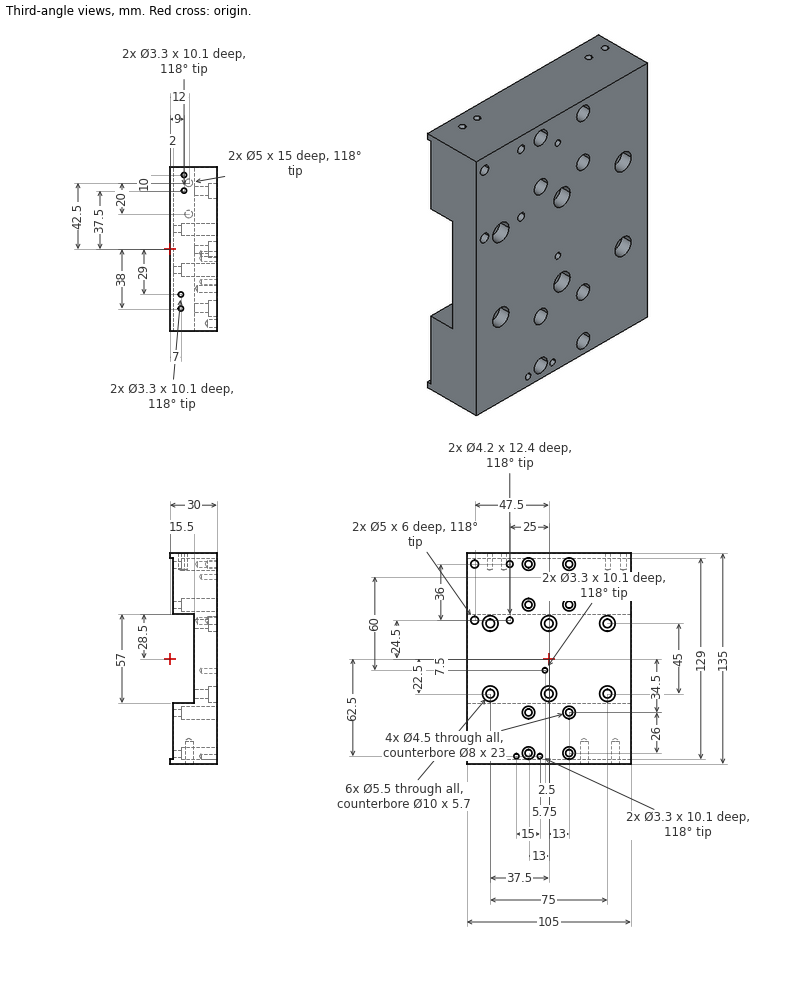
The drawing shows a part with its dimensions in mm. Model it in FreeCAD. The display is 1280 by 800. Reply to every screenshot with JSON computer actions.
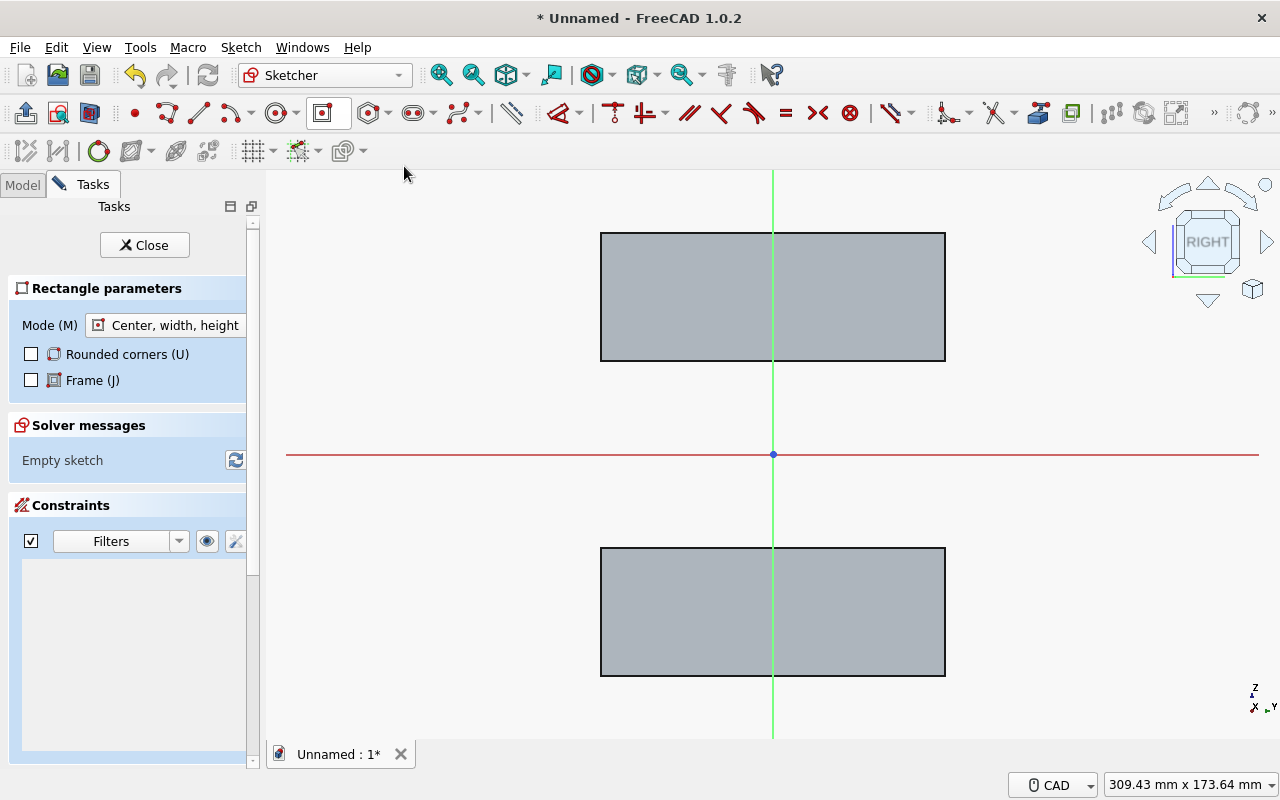
{"action": "left_click", "coordinate": [773, 454]}
{"action": "left_click", "coordinate": [945, 243]}
{"action": "key", "text": "Escape"}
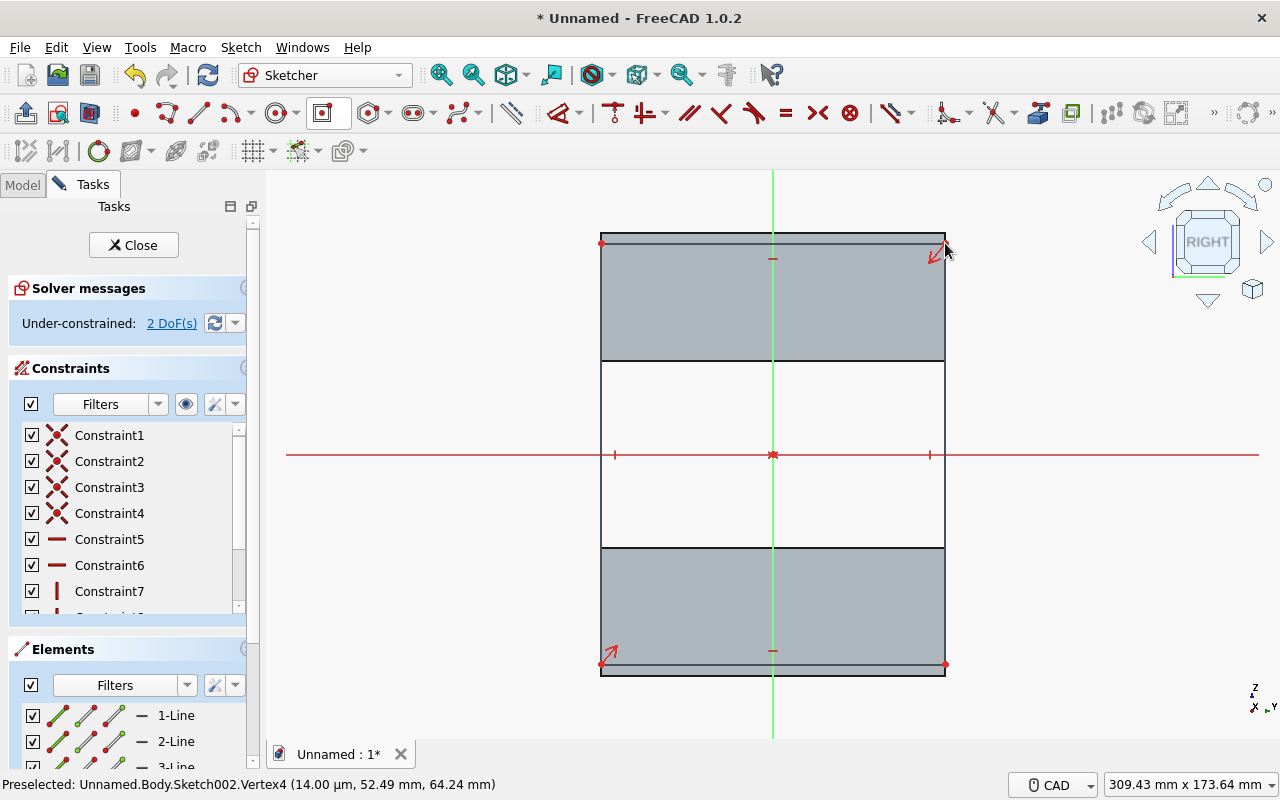
{"action": "left_click", "coordinate": [558, 114]}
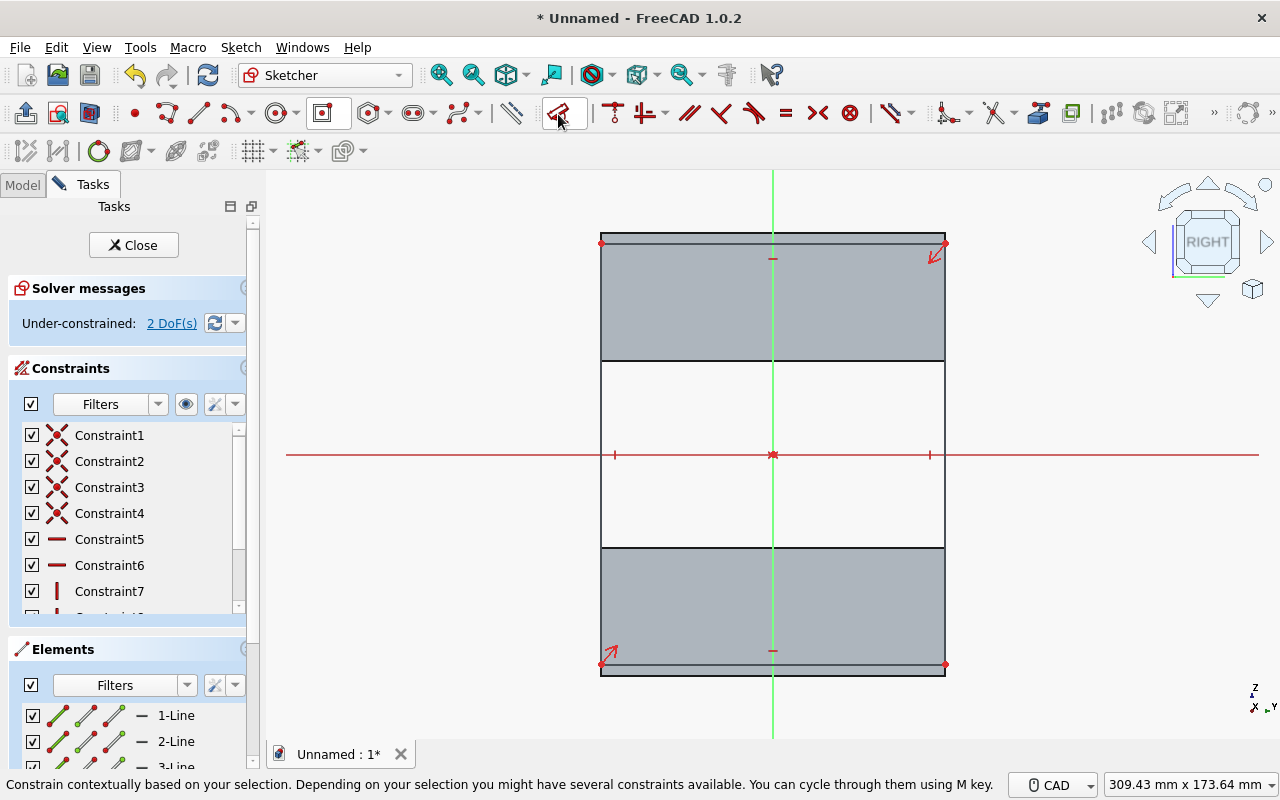
{"action": "left_click", "coordinate": [704, 665]}
{"action": "left_click", "coordinate": [694, 699]}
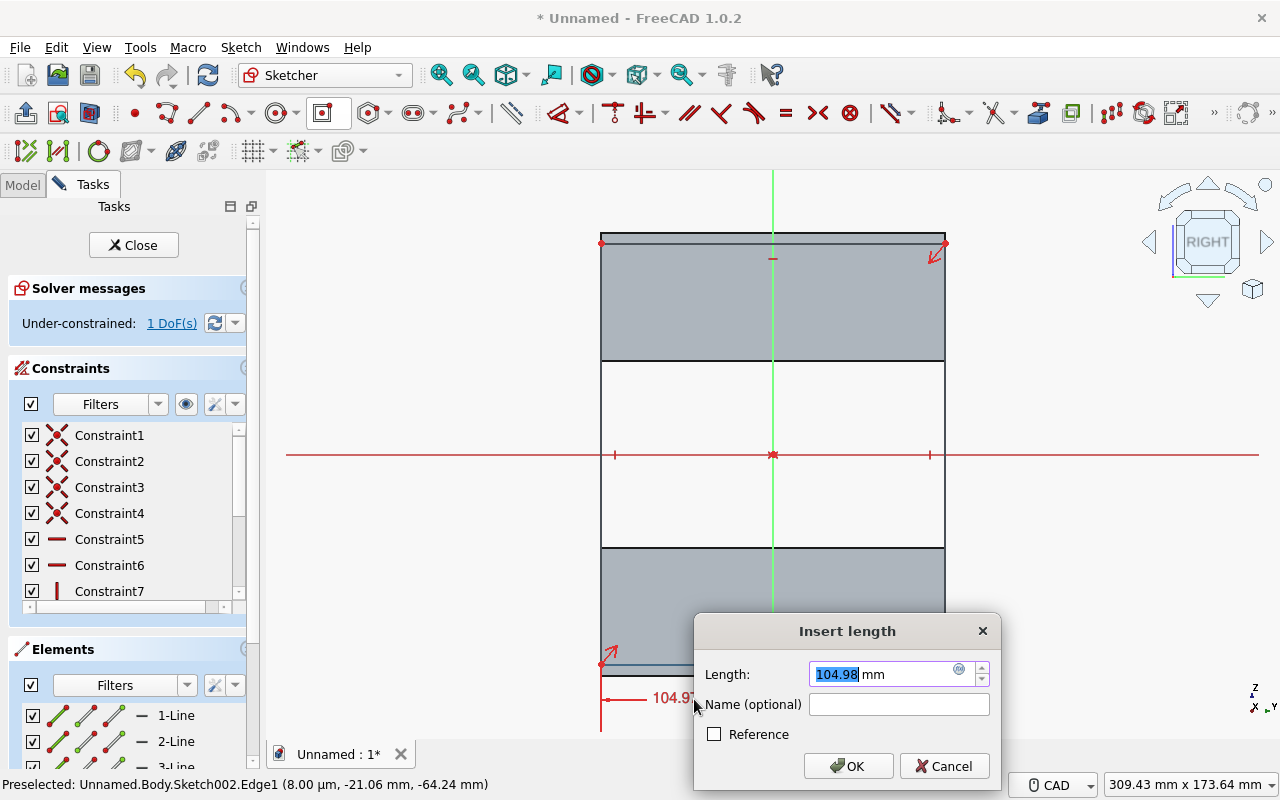
{"action": "type", "text": "105"}
{"action": "key", "text": "Return"}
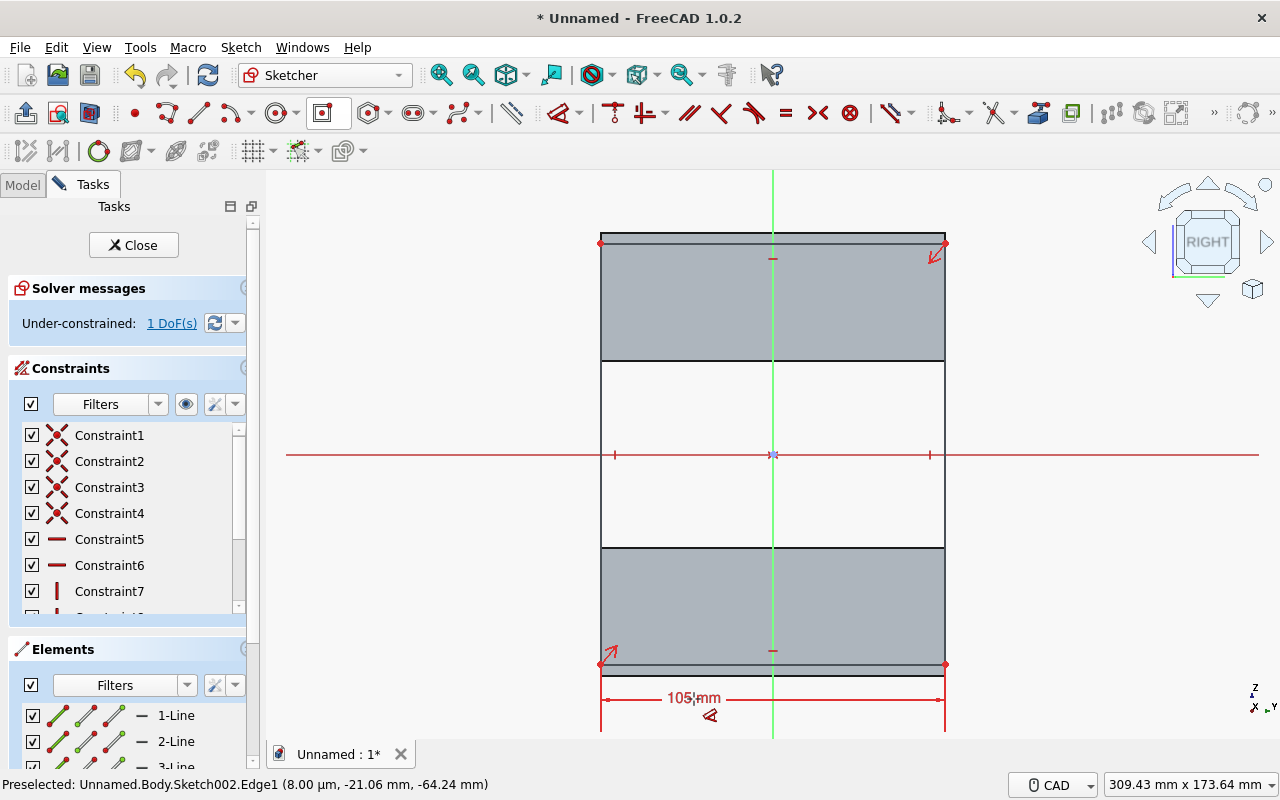
{"action": "left_click", "coordinate": [945, 539]}
{"action": "left_click", "coordinate": [979, 358]}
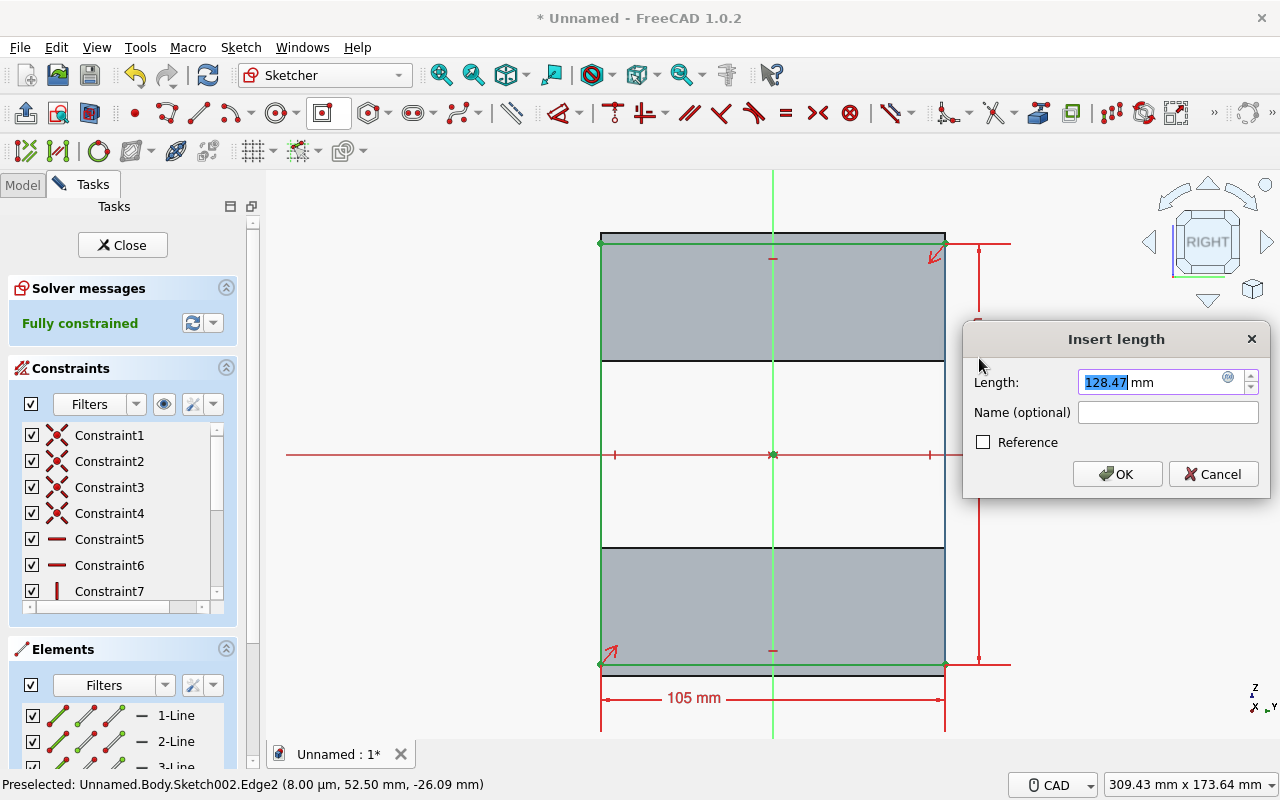
{"action": "type", "text": "129"}
{"action": "key", "text": "Return"}
{"action": "key", "text": "Escape"}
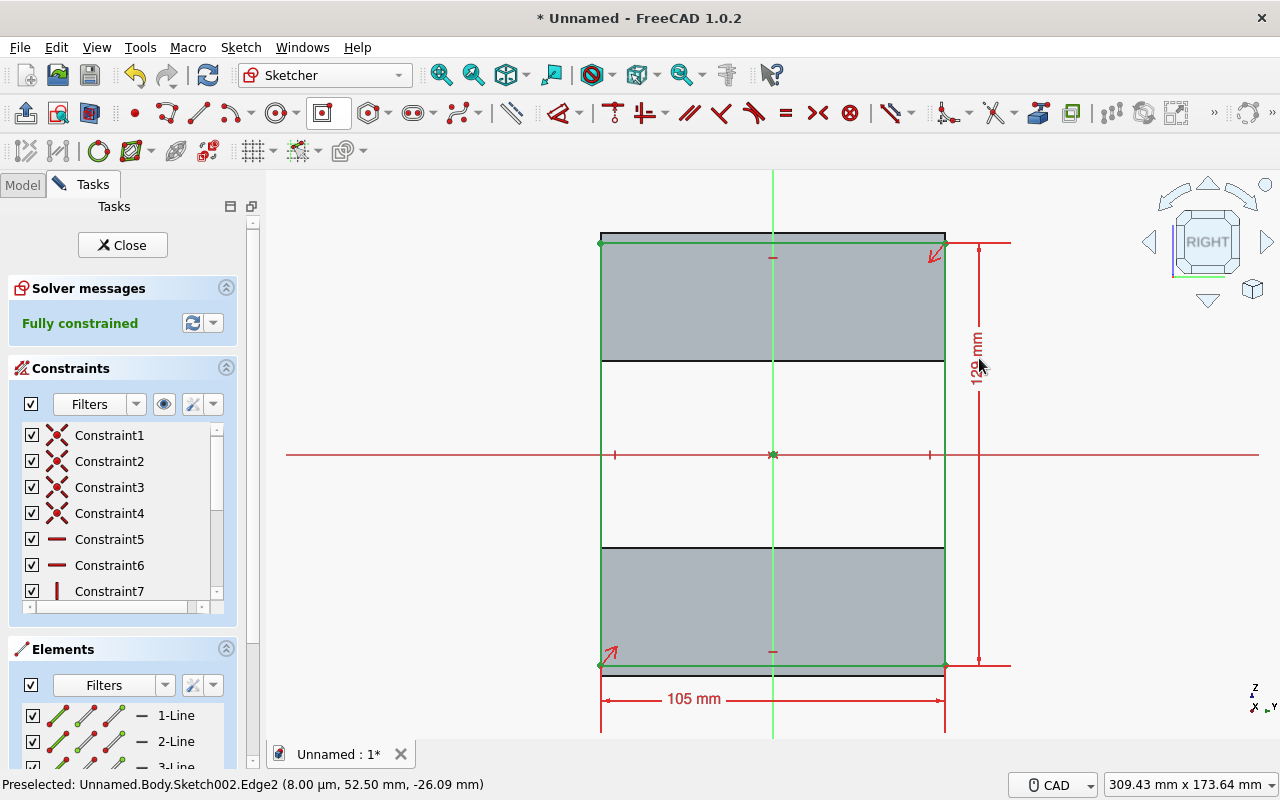
{"action": "left_click", "coordinate": [123, 245]}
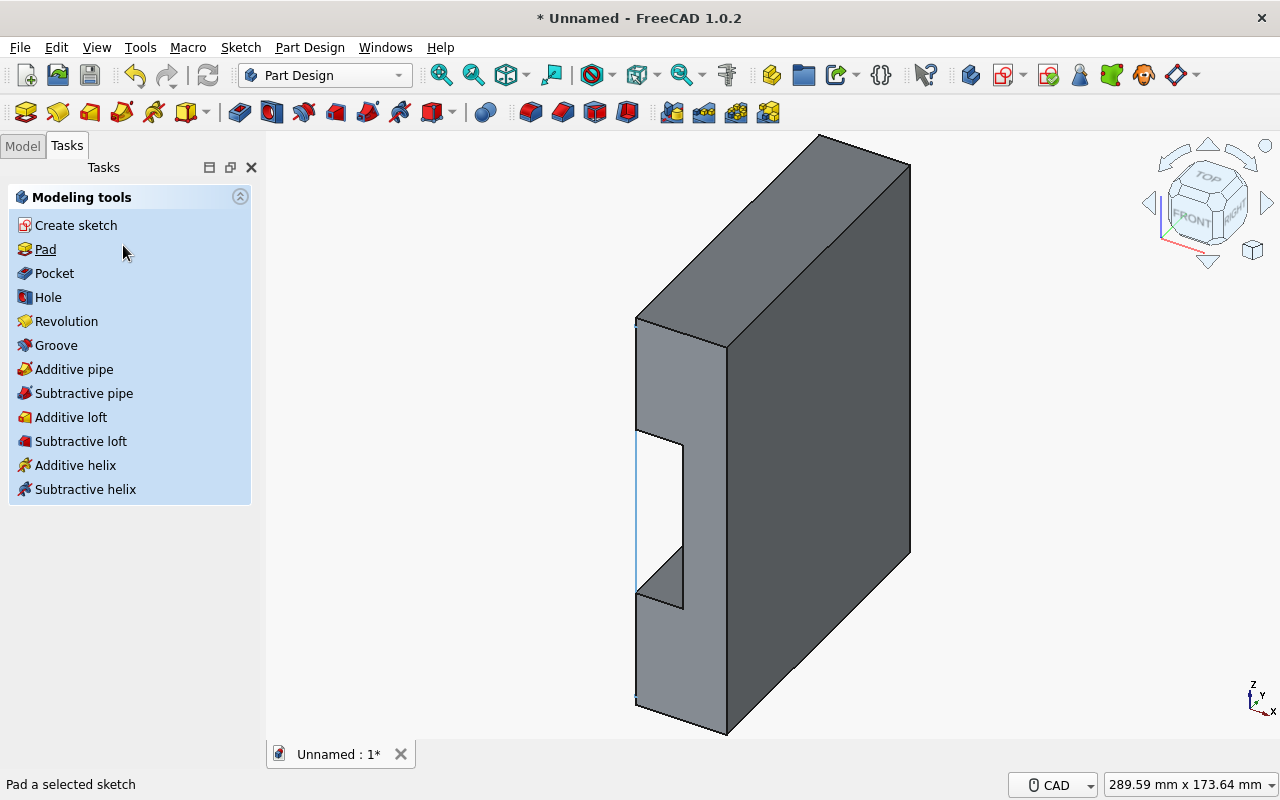
{"action": "left_click", "coordinate": [240, 112]}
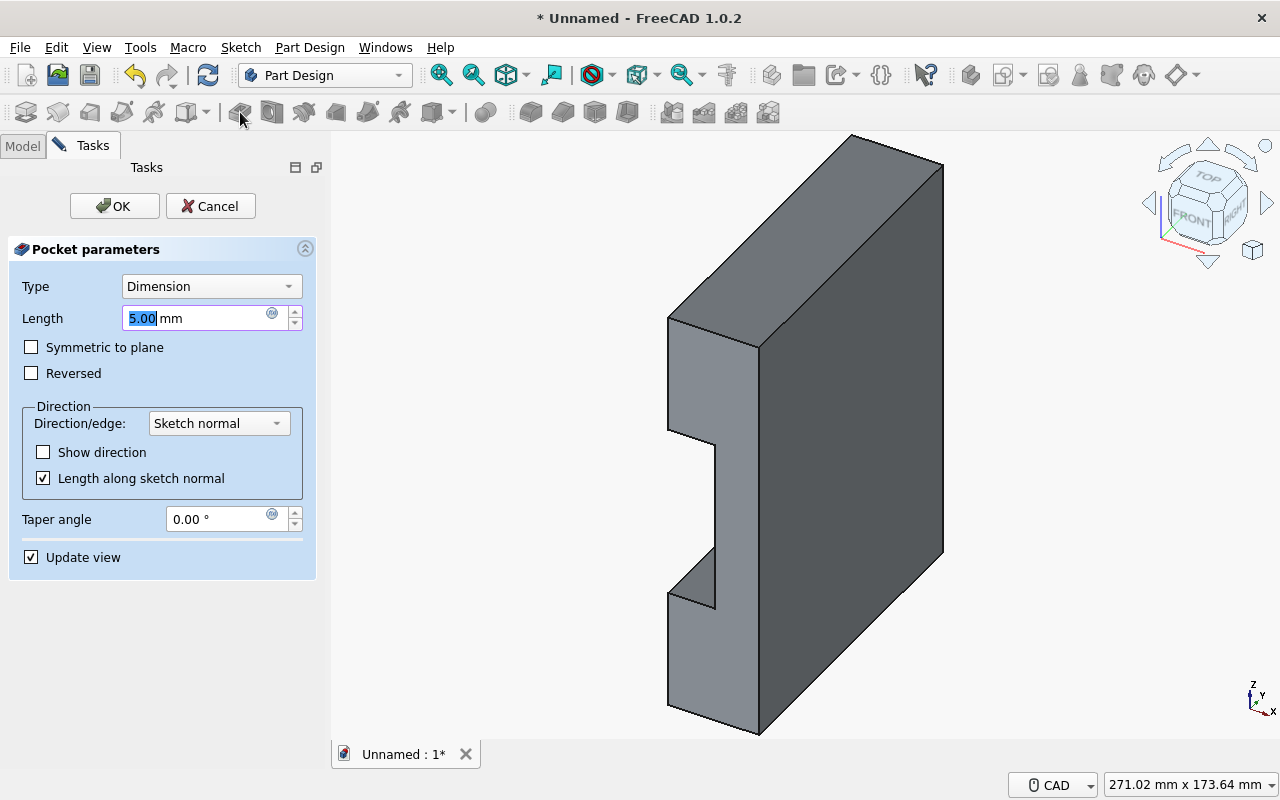
{"action": "type", "text": "2"}
{"action": "key", "text": "Tab"}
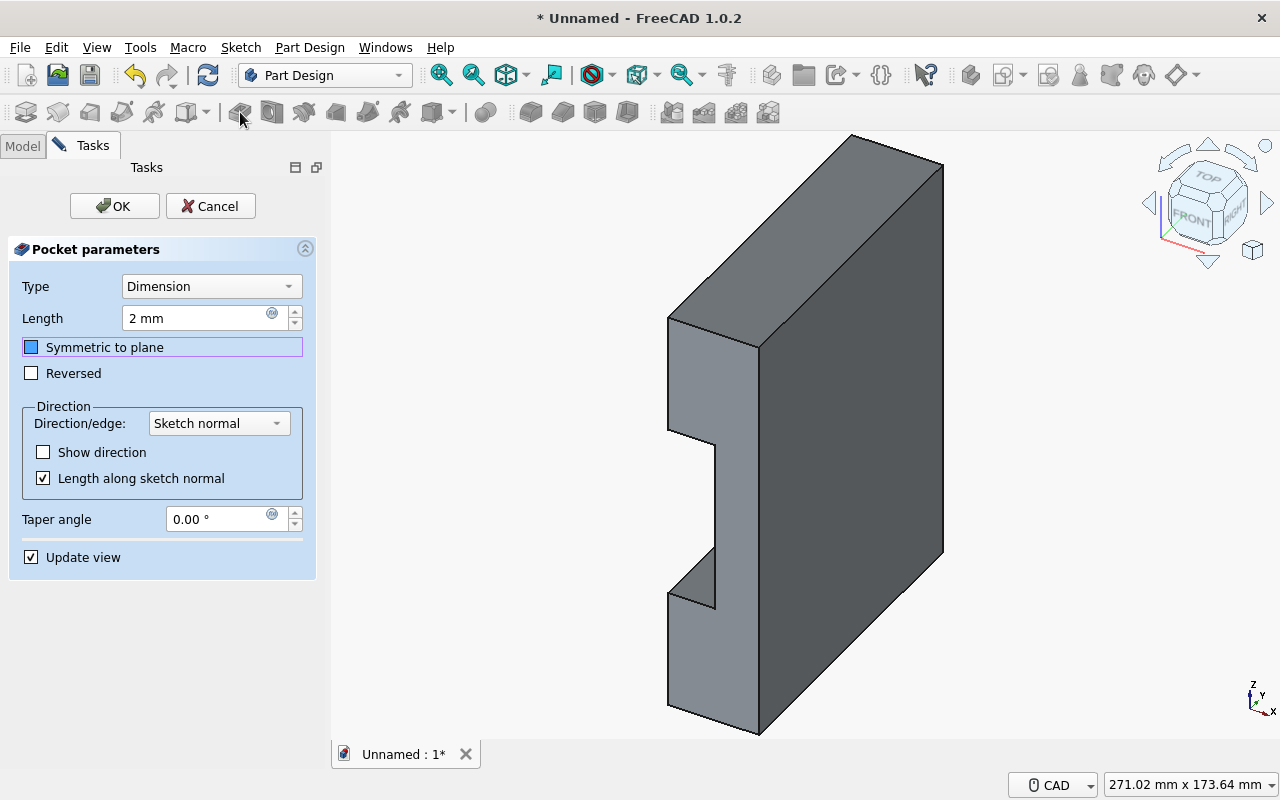
{"action": "left_click", "coordinate": [30, 373]}